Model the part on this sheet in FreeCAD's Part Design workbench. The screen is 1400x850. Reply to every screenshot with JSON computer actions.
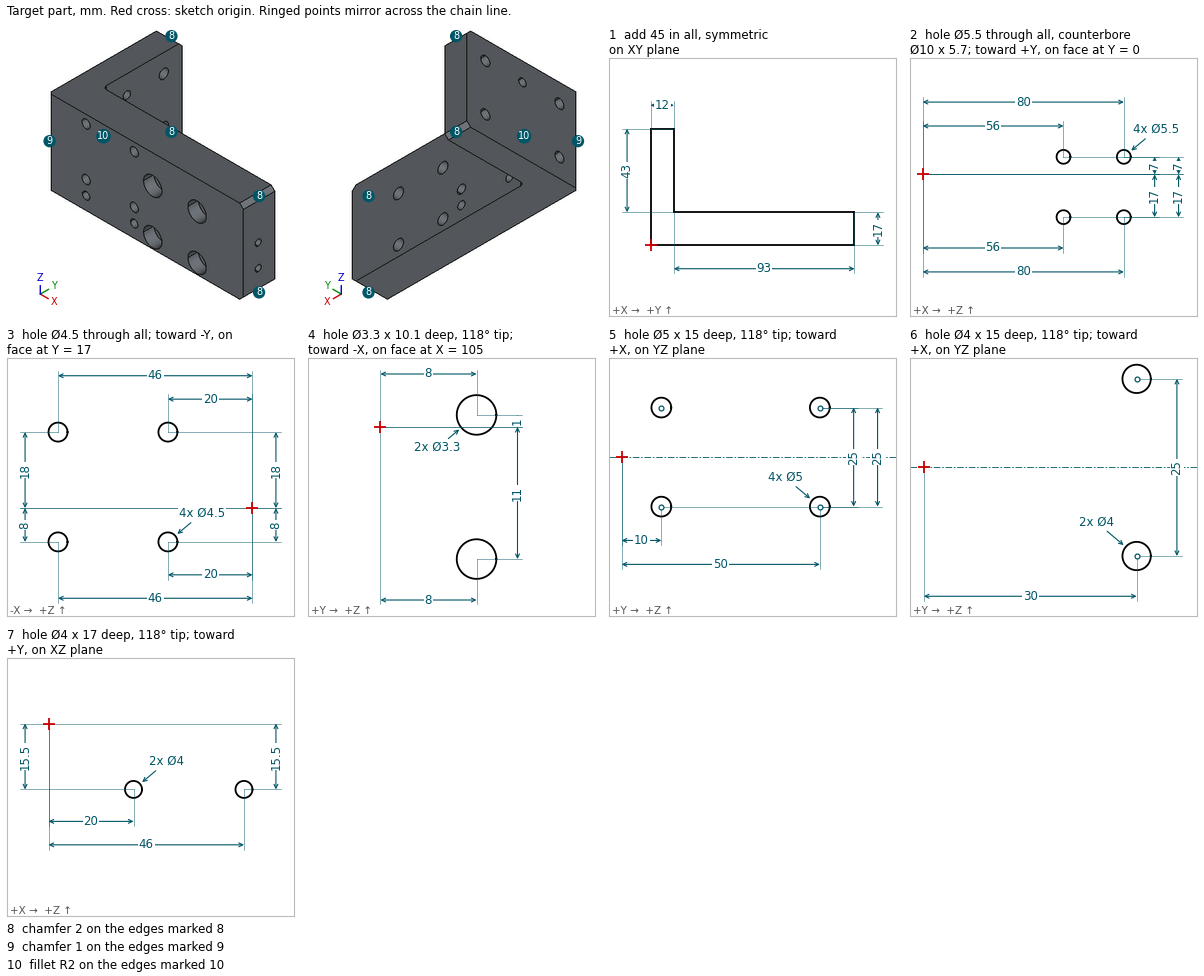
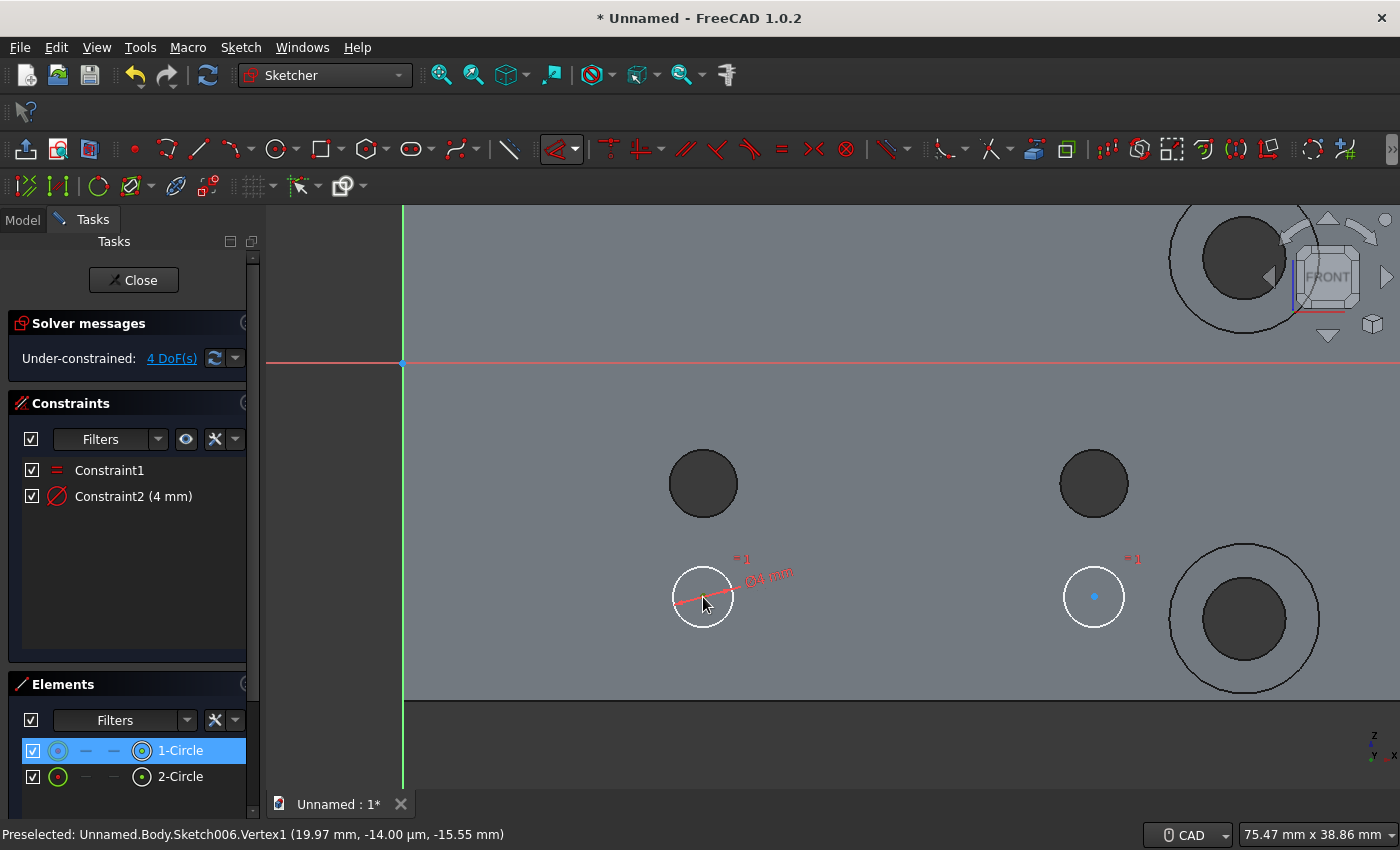
{"action": "key", "text": "l"}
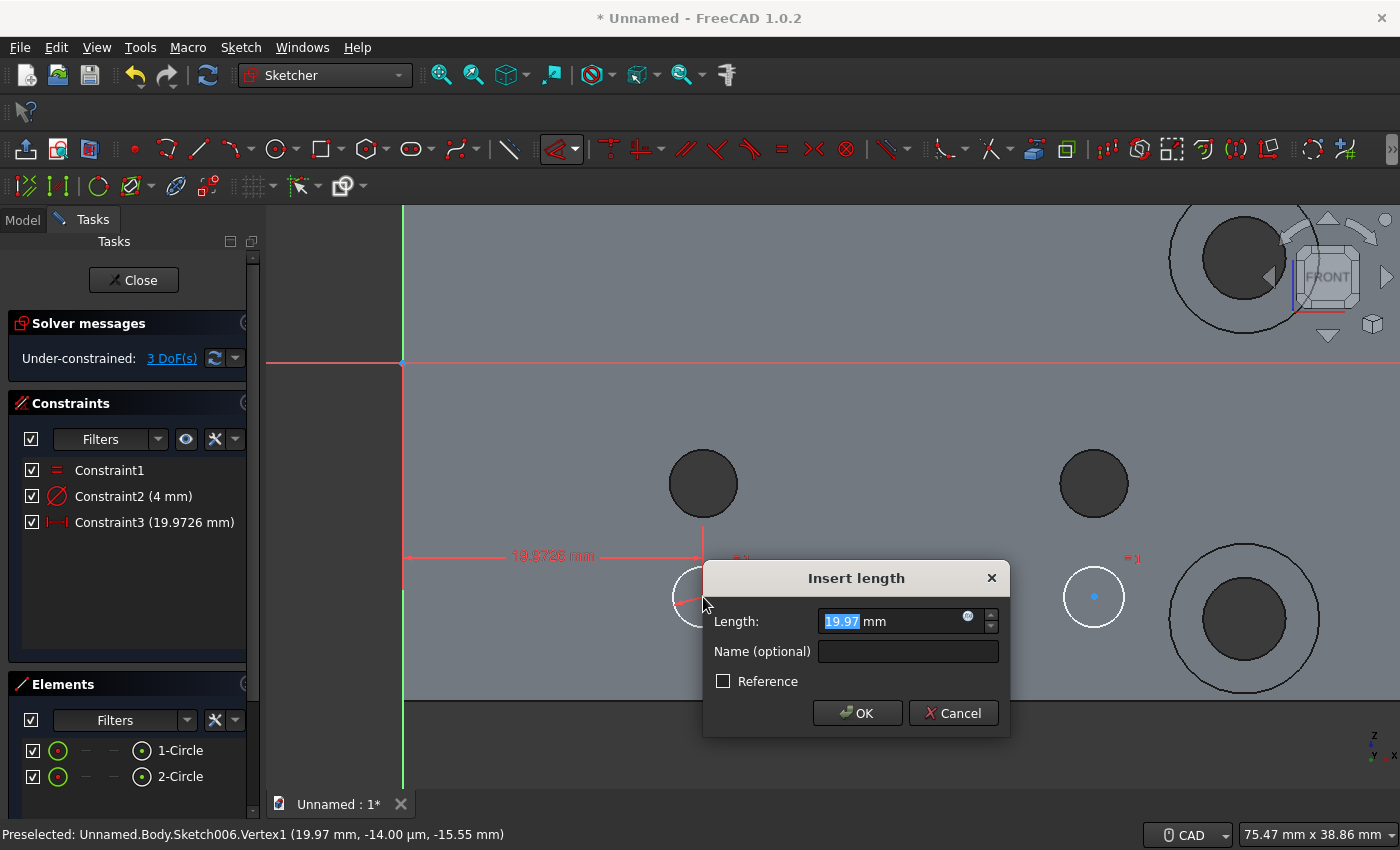
{"action": "type", "text": "20"}
{"action": "key", "text": "Return"}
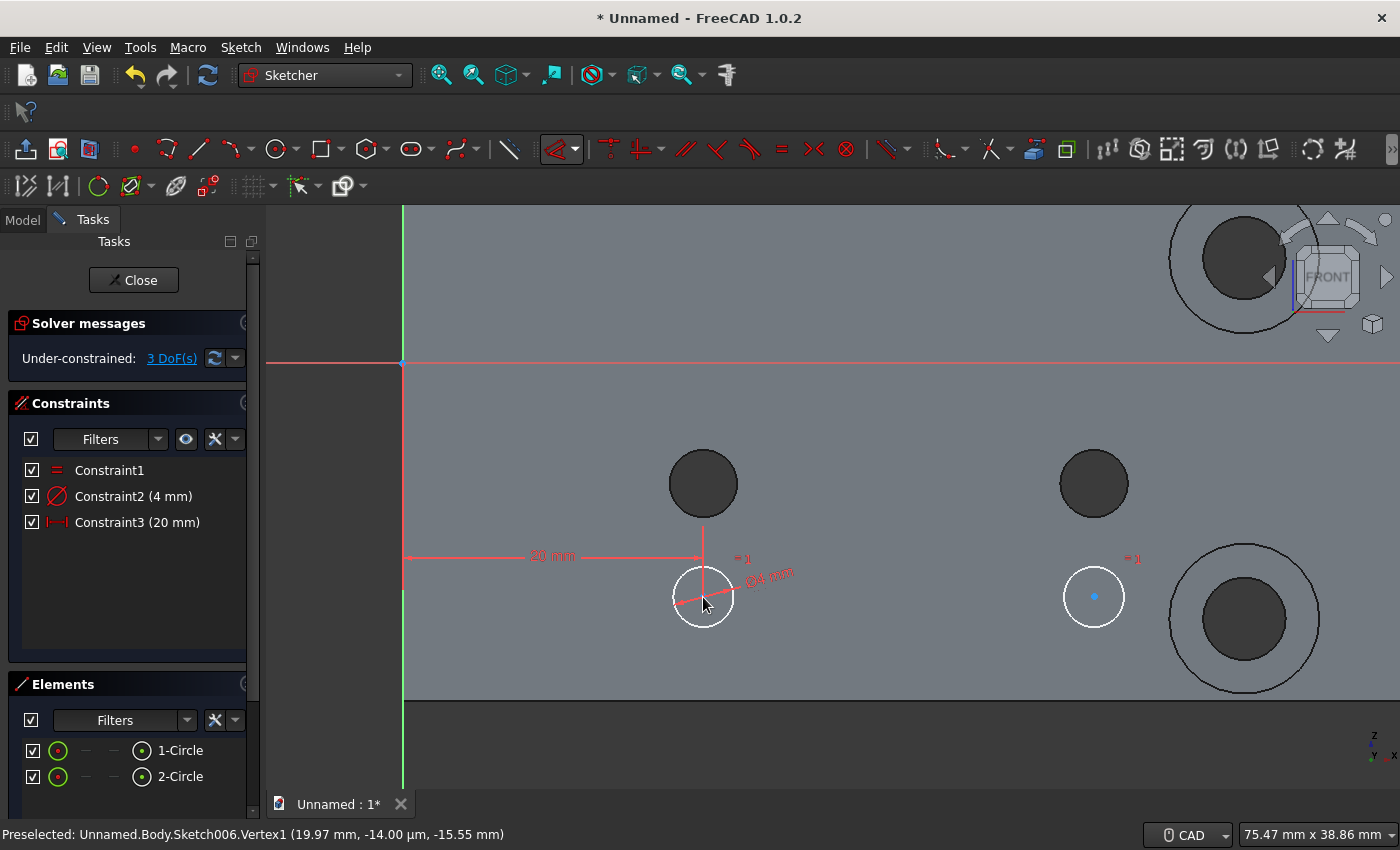
{"action": "left_click", "coordinate": [1094, 597]}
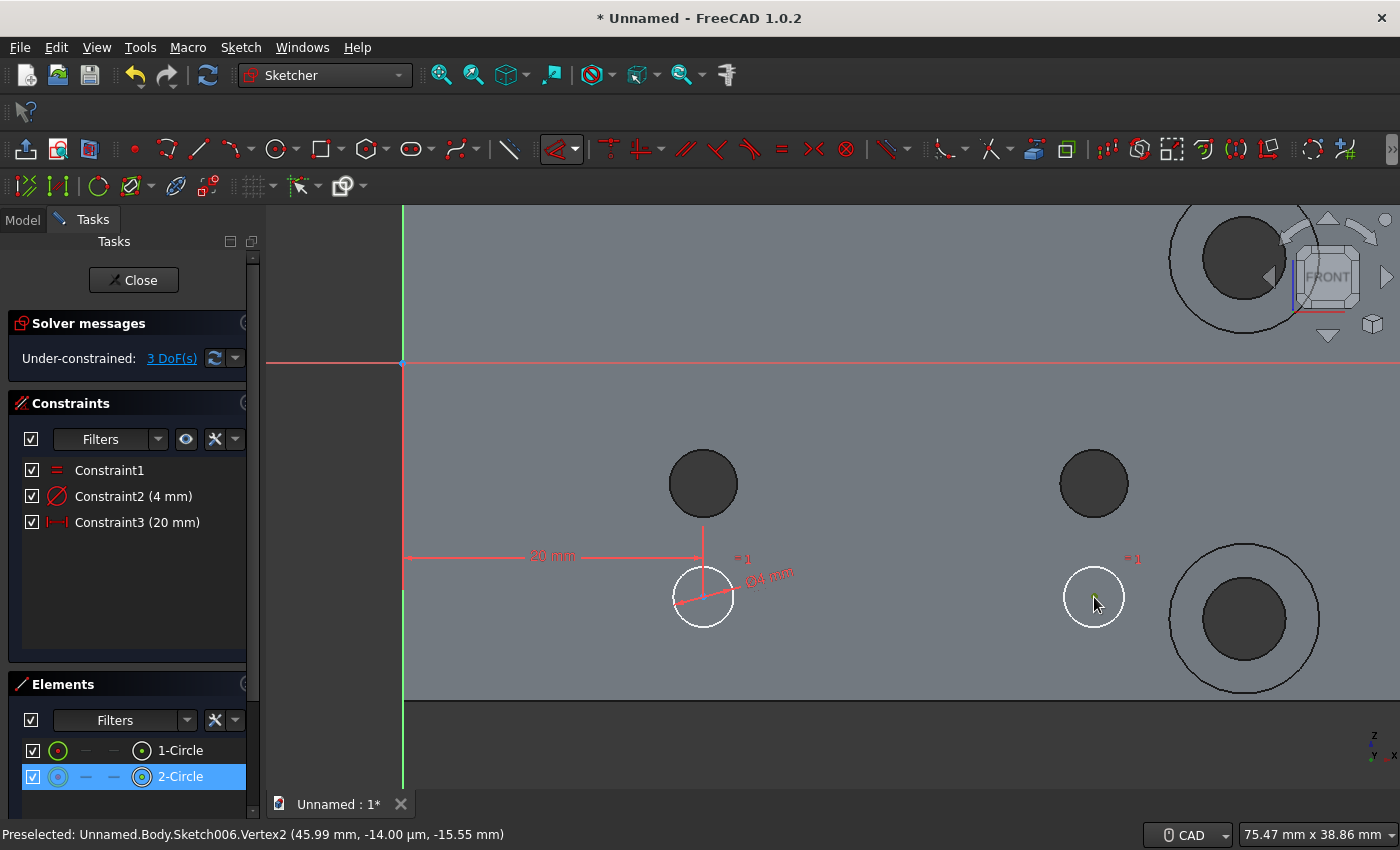
{"action": "key", "text": "l"}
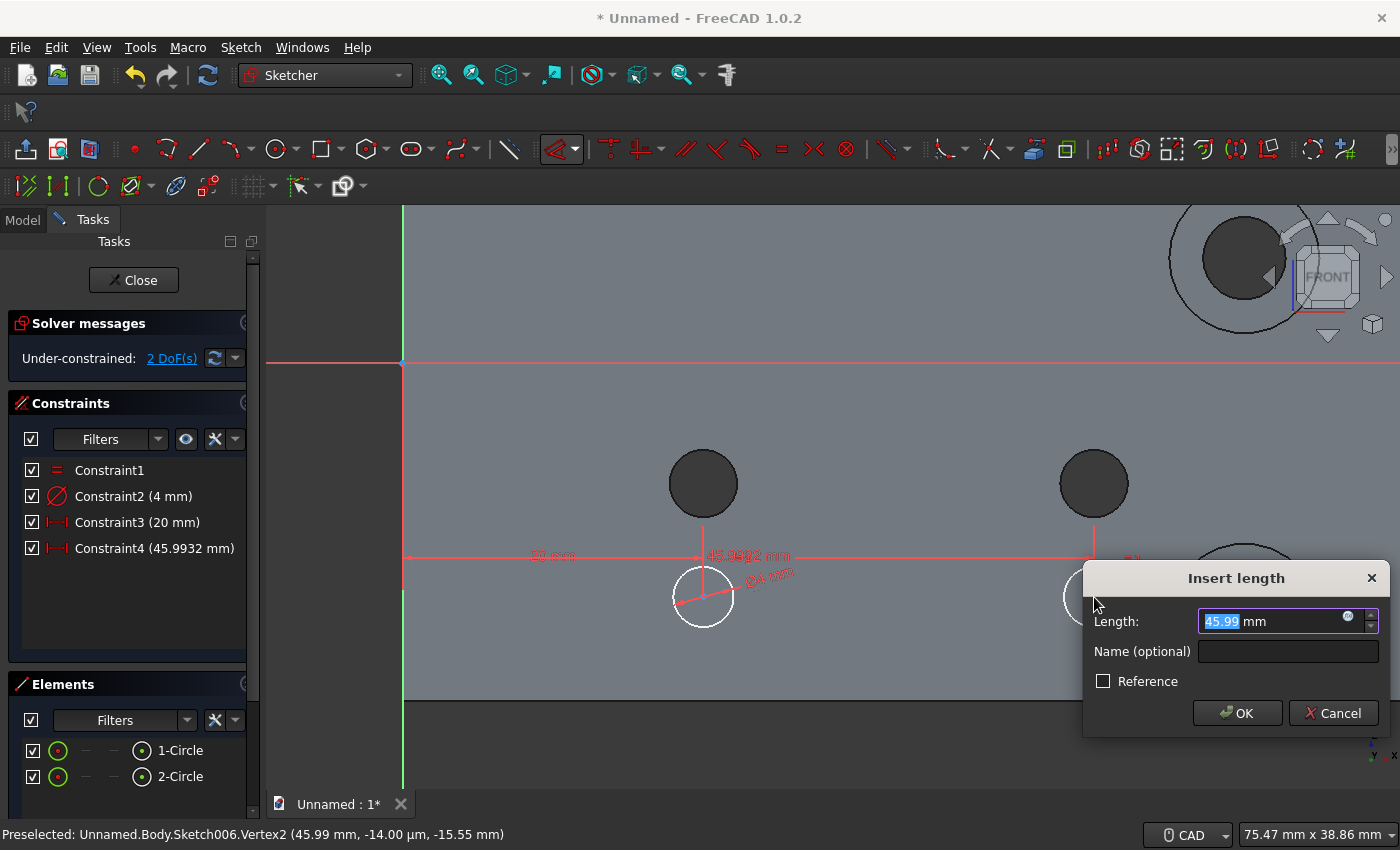
{"action": "type", "text": "46"}
{"action": "key", "text": "Return"}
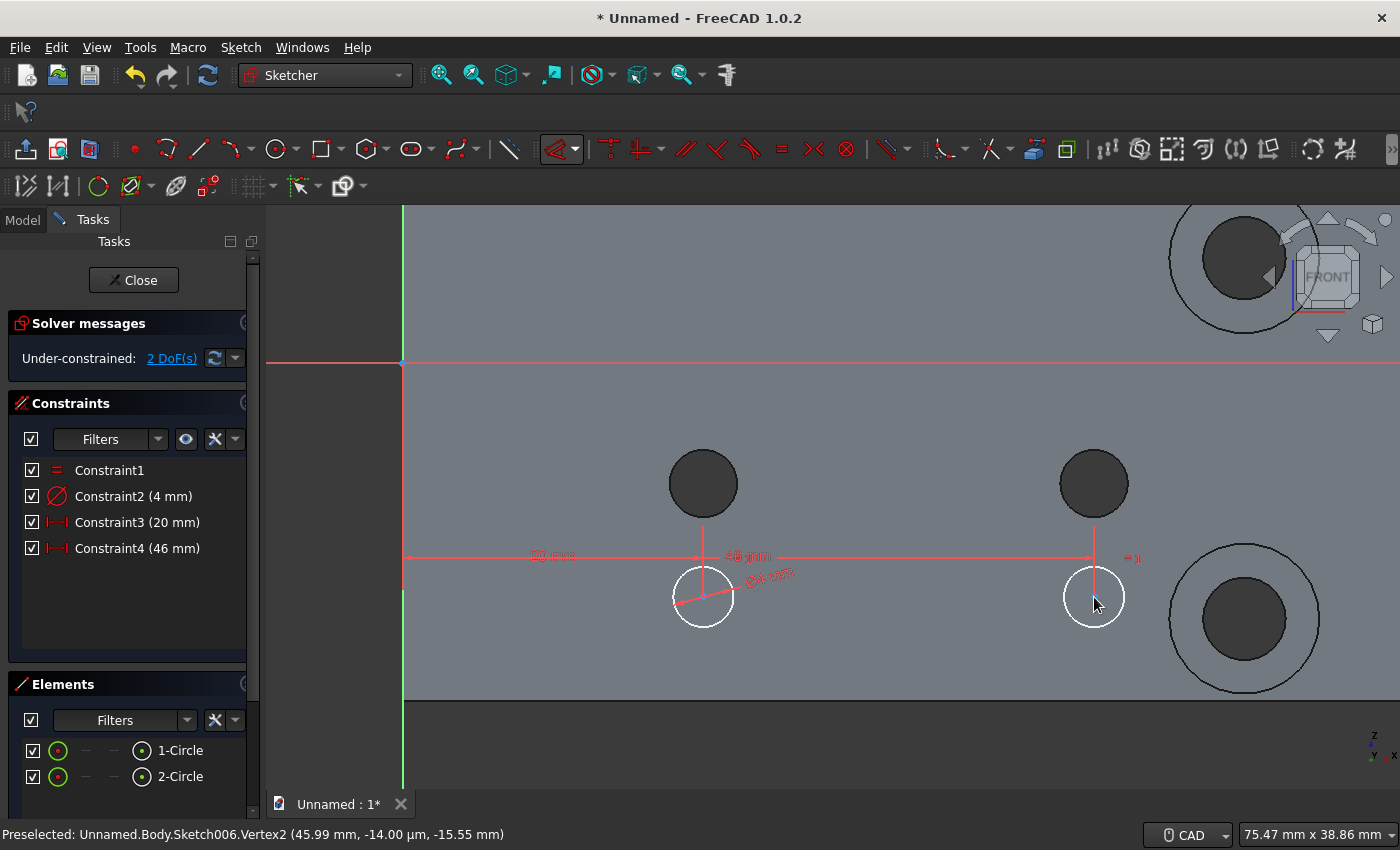
{"action": "left_click", "coordinate": [703, 597]}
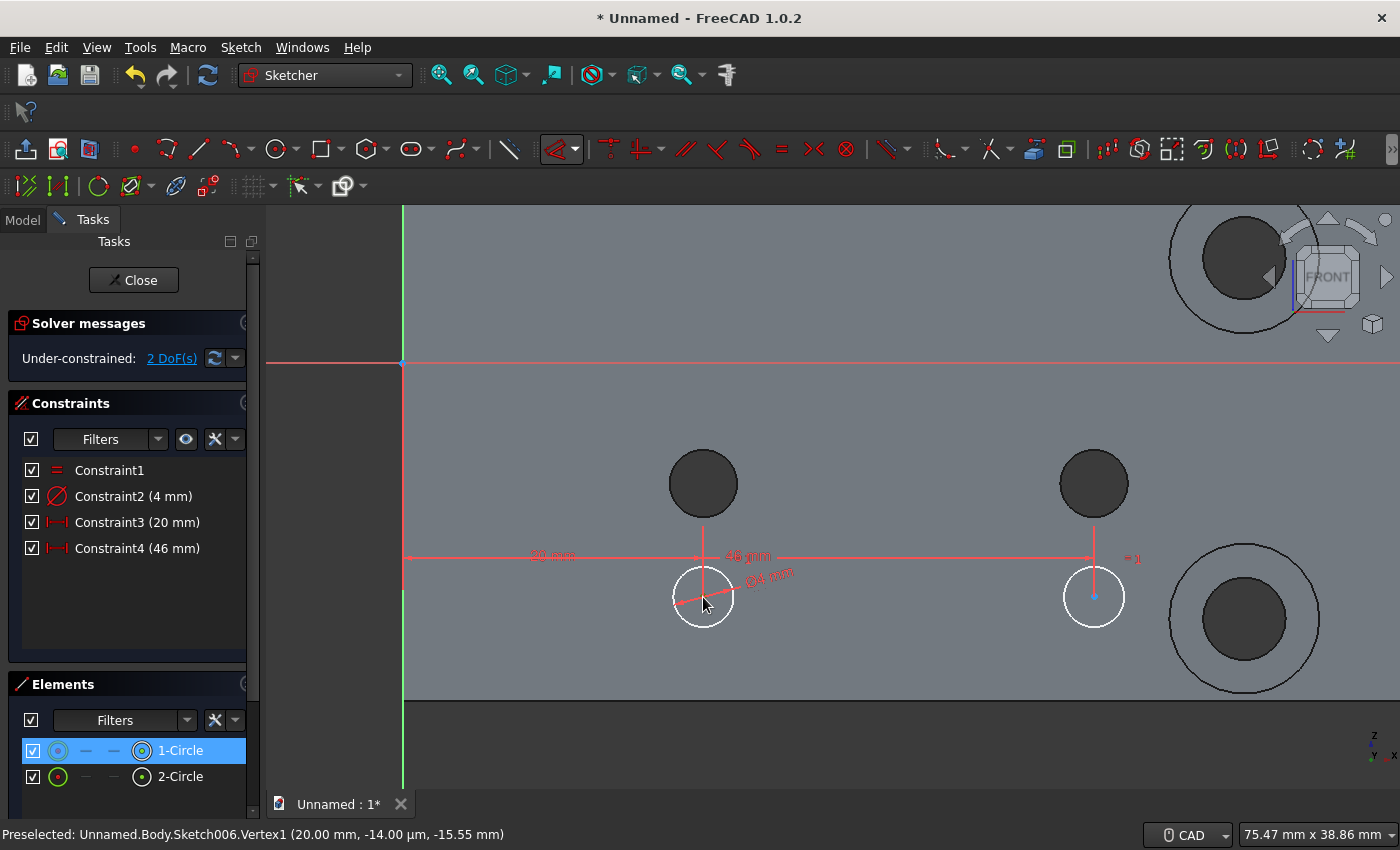
{"action": "key", "text": "i"}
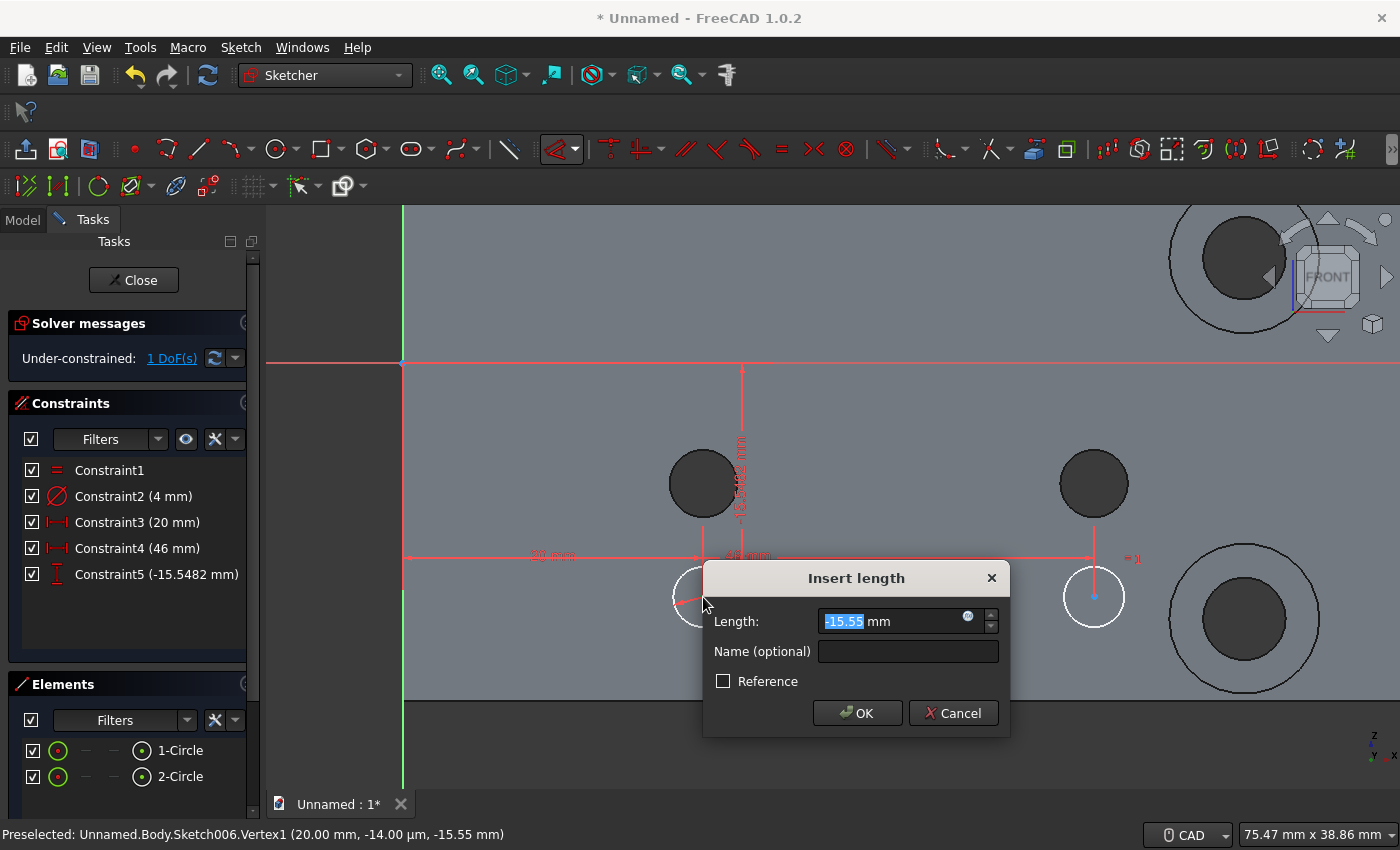
{"action": "type", "text": "-15.5"}
{"action": "key", "text": "Return"}